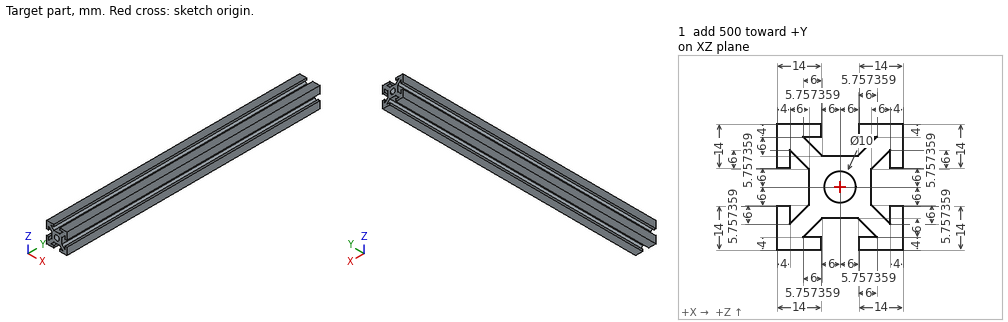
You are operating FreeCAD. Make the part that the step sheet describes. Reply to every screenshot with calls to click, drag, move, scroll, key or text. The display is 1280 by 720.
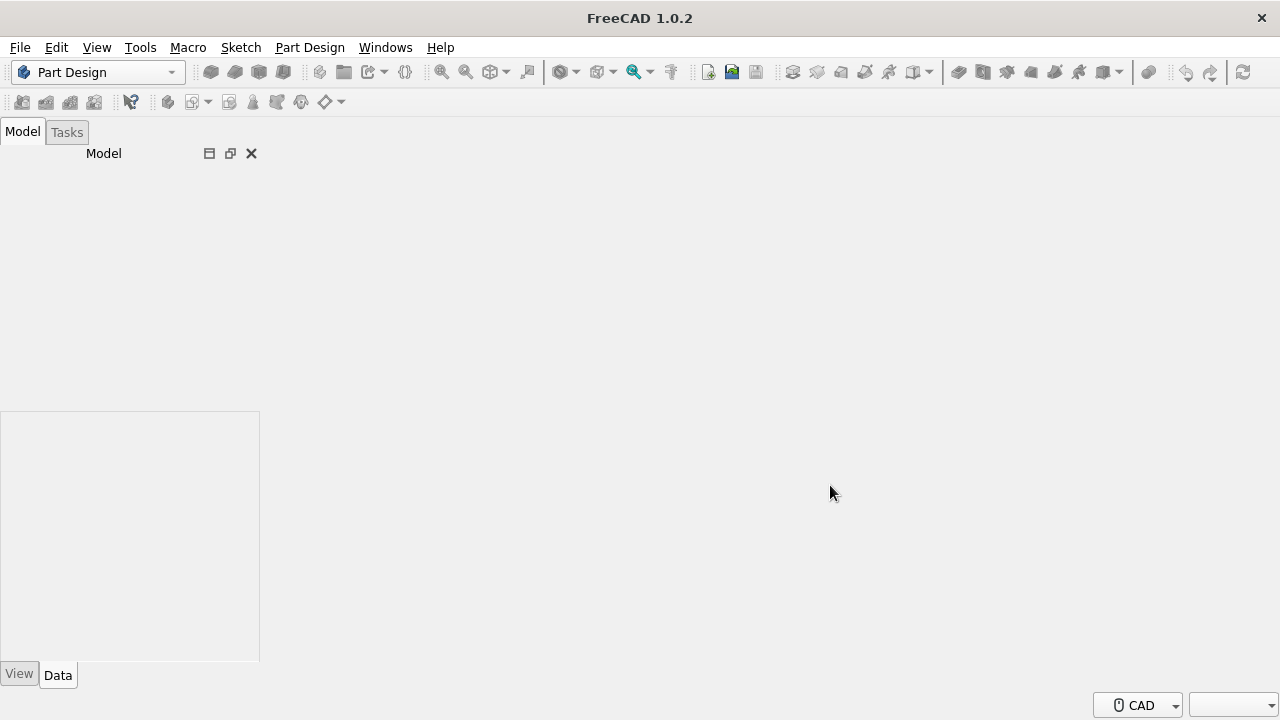
click(708, 72)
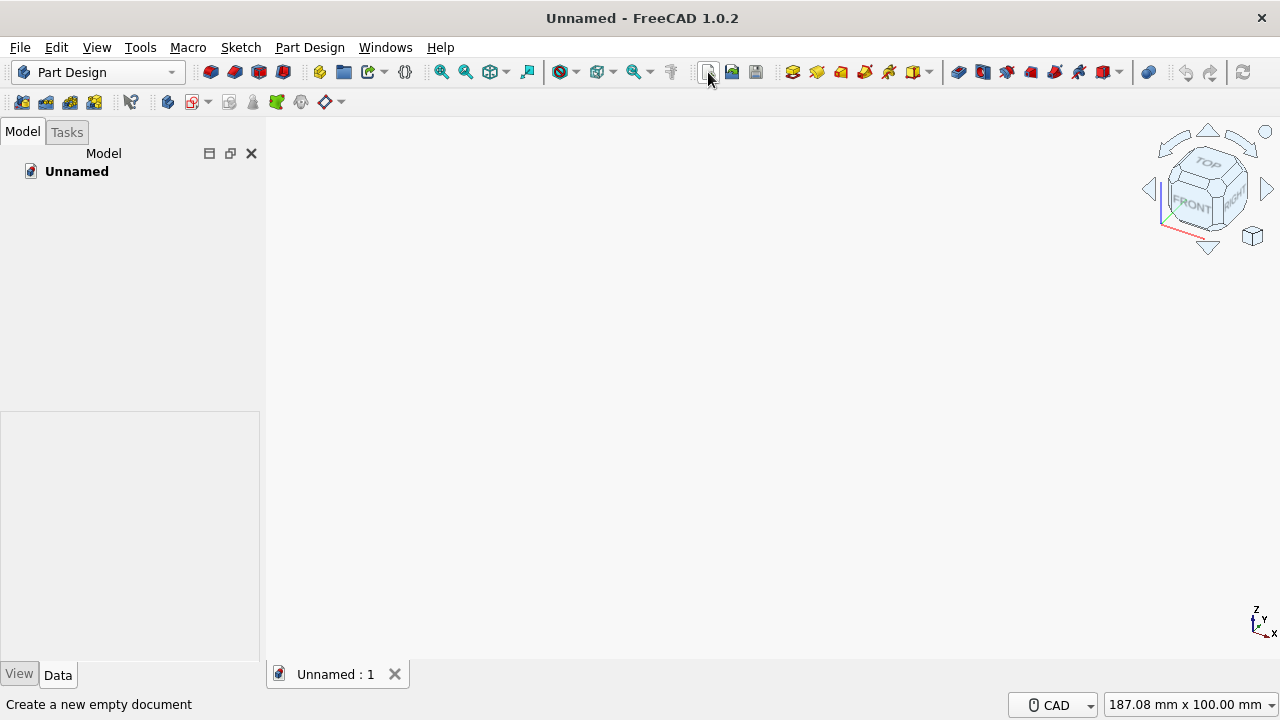
click(192, 102)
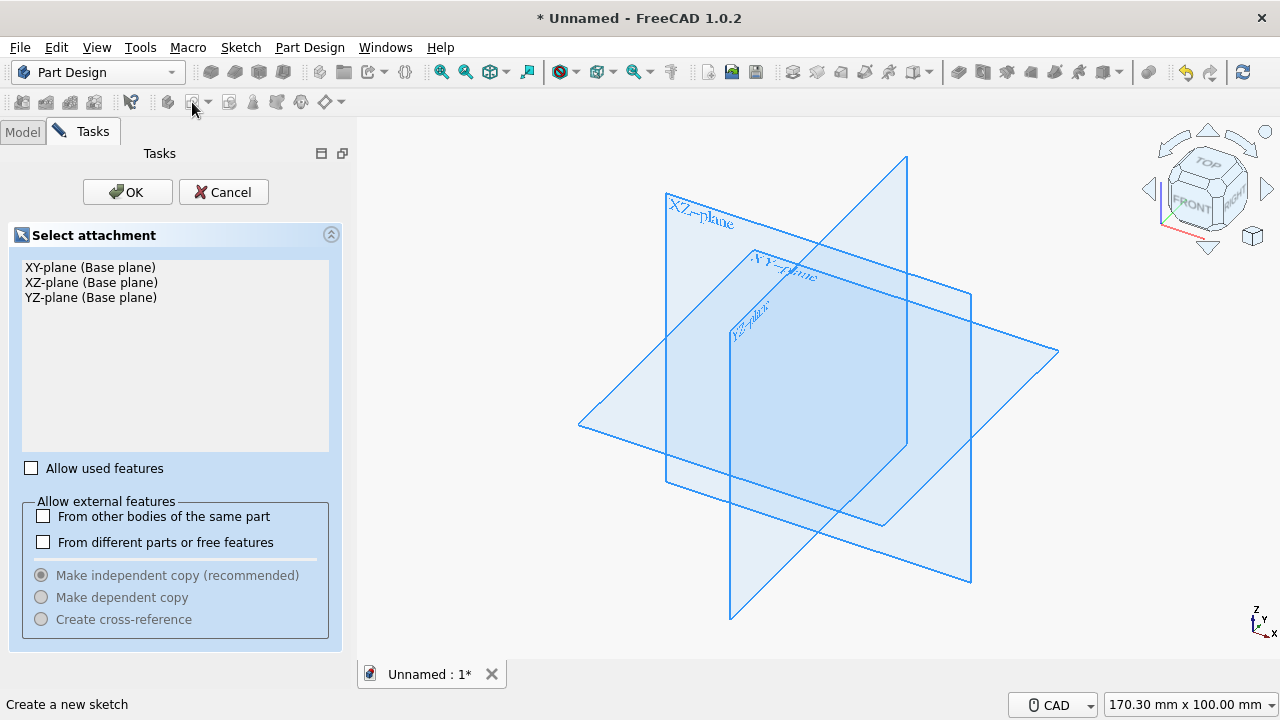
click(82, 282)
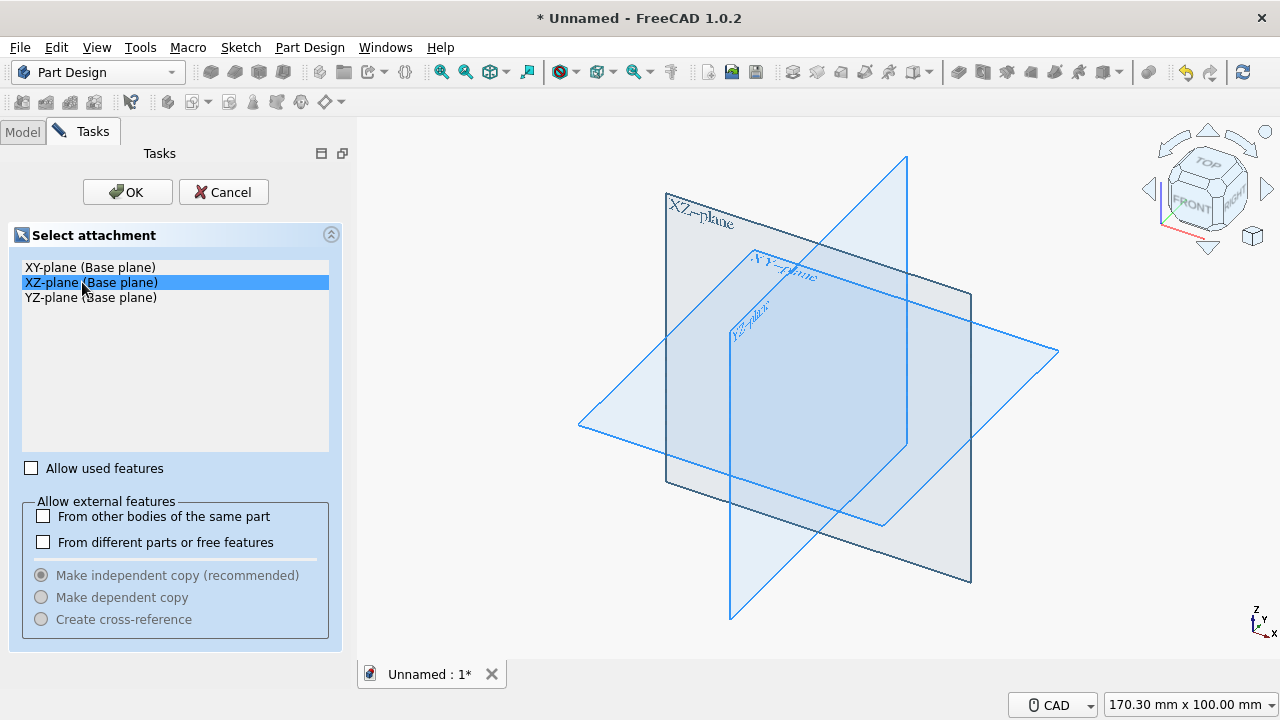
click(128, 192)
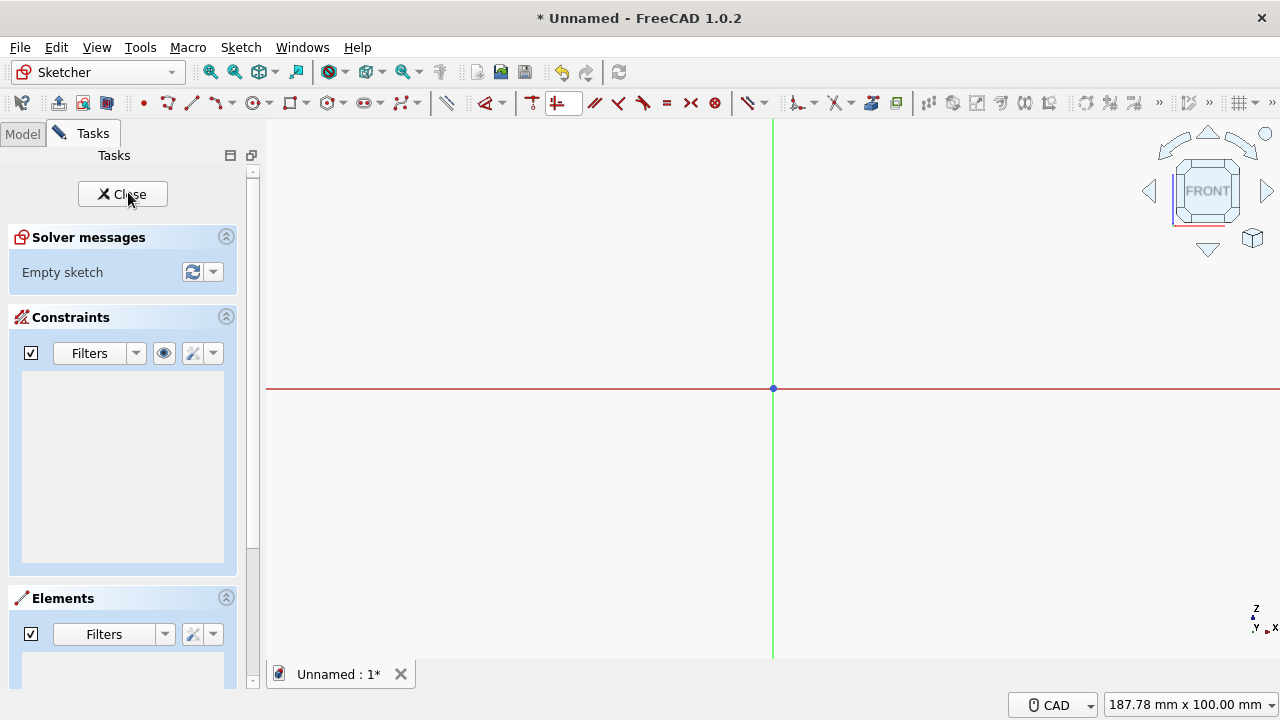
scroll(912, 389, up, 2)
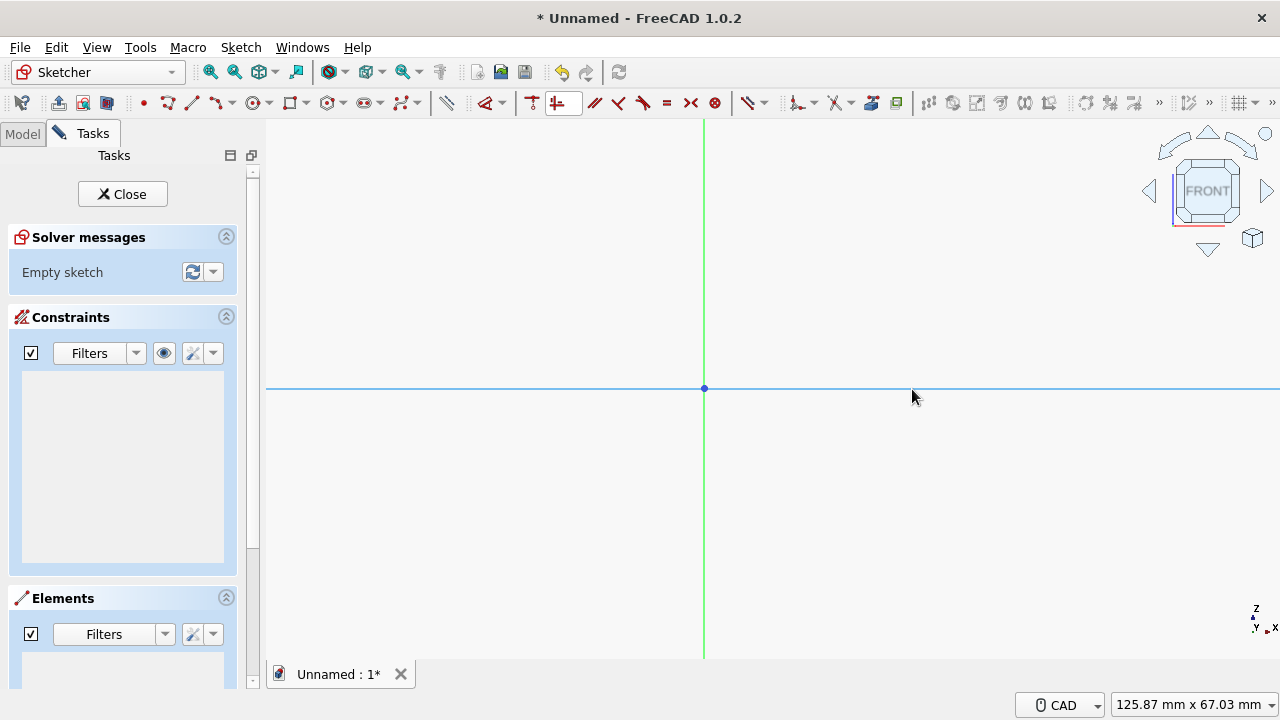
click(168, 104)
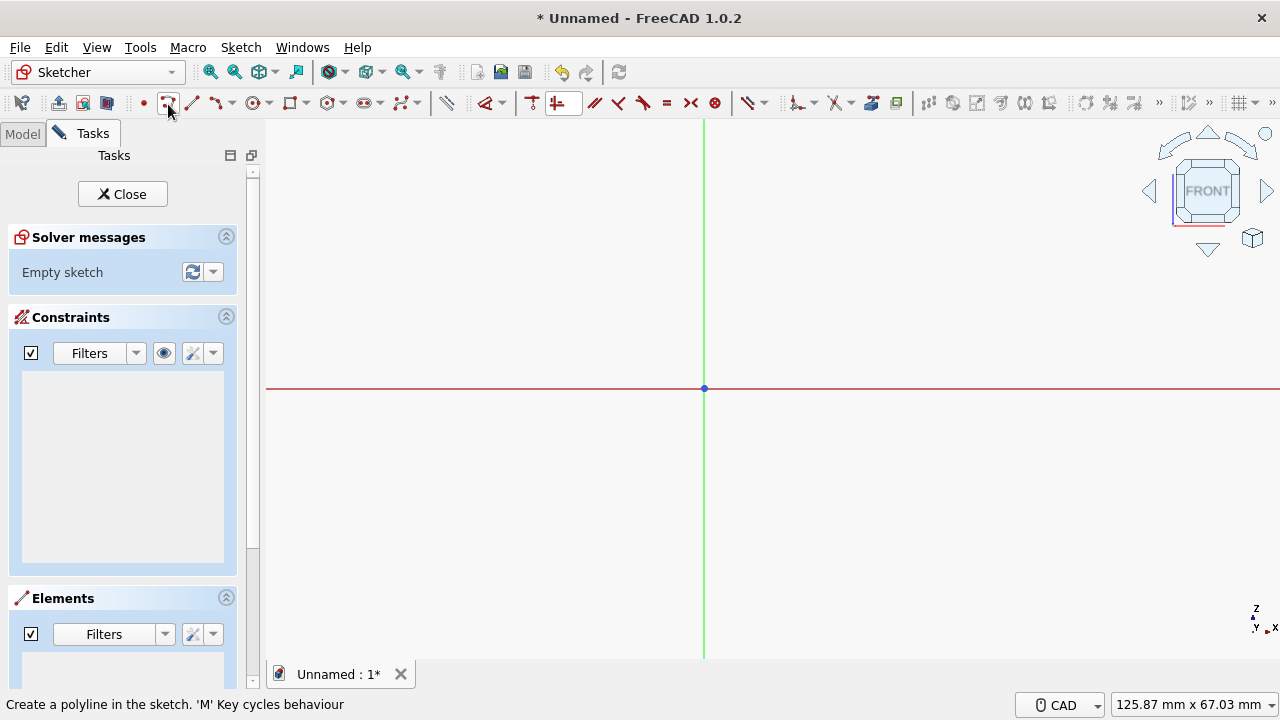
click(624, 435)
click(624, 342)
click(575, 294)
click(575, 340)
click(543, 340)
click(543, 228)
click(656, 228)
click(656, 260)
click(610, 260)
click(658, 308)
click(751, 308)
click(799, 260)
click(753, 260)
click(753, 228)
click(865, 228)
click(865, 340)
click(833, 340)
click(833, 294)
click(785, 342)
click(785, 435)
click(833, 483)
click(833, 437)
click(865, 437)
click(865, 550)
click(753, 550)
click(753, 518)
click(799, 518)
click(751, 469)
click(658, 469)
click(610, 518)
click(656, 518)
click(656, 550)
click(543, 550)
click(543, 437)
click(575, 437)
click(575, 483)
click(624, 436)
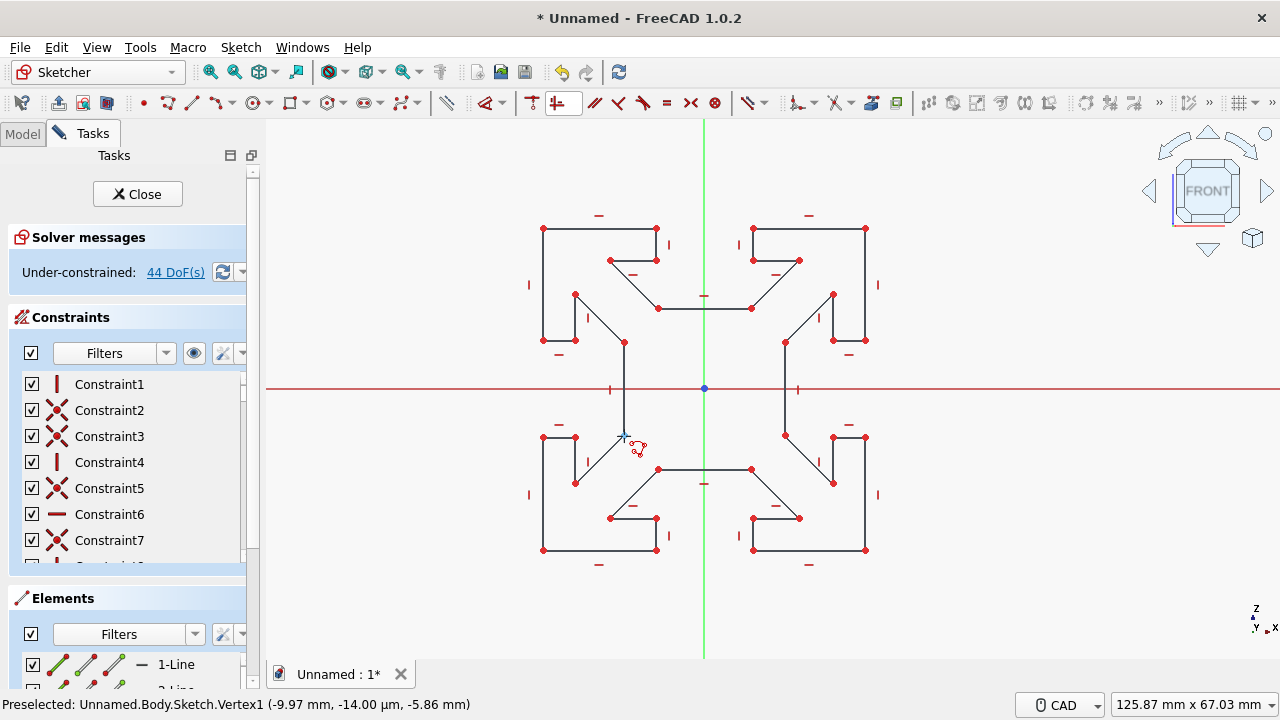
click(254, 104)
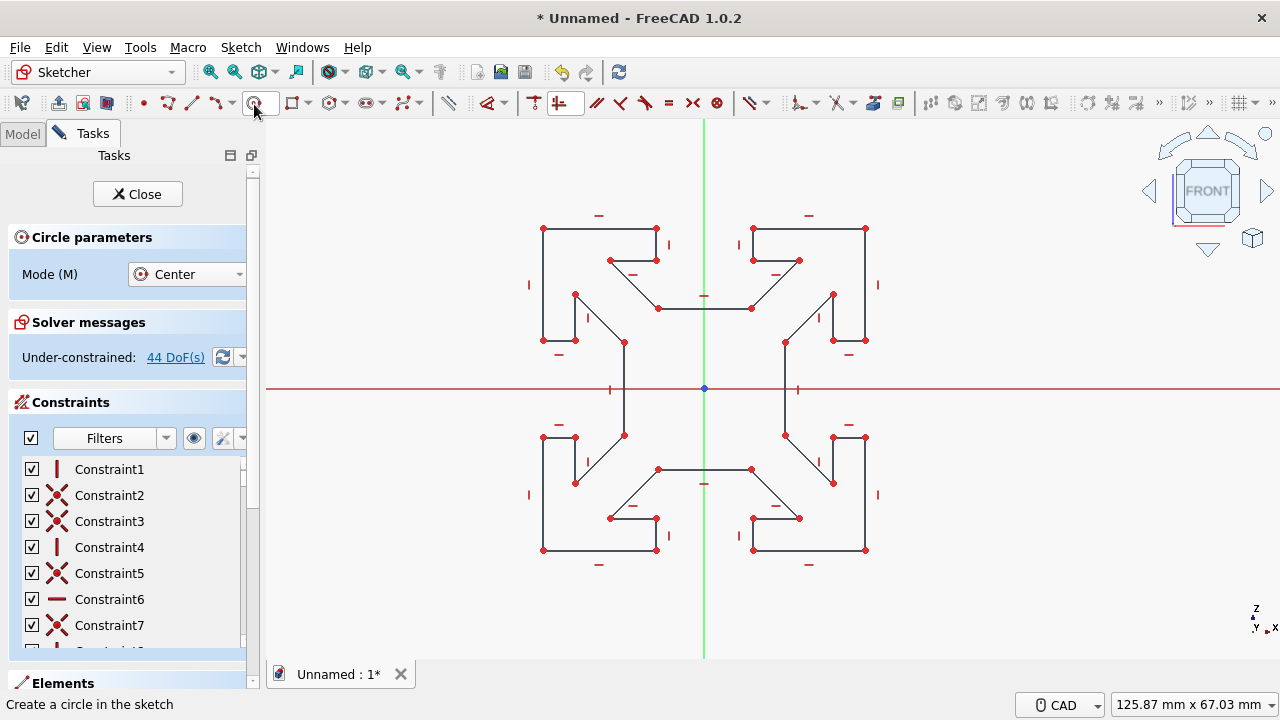
click(704, 389)
click(733, 360)
key(Escape)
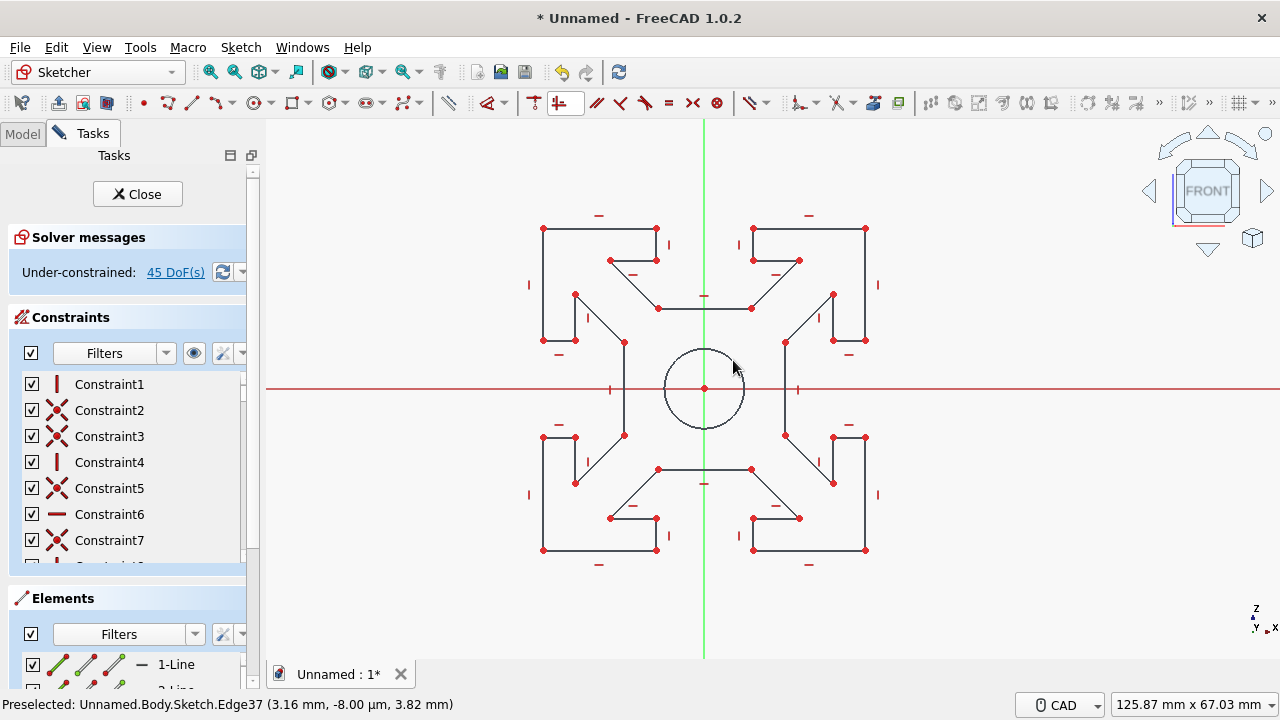
click(488, 104)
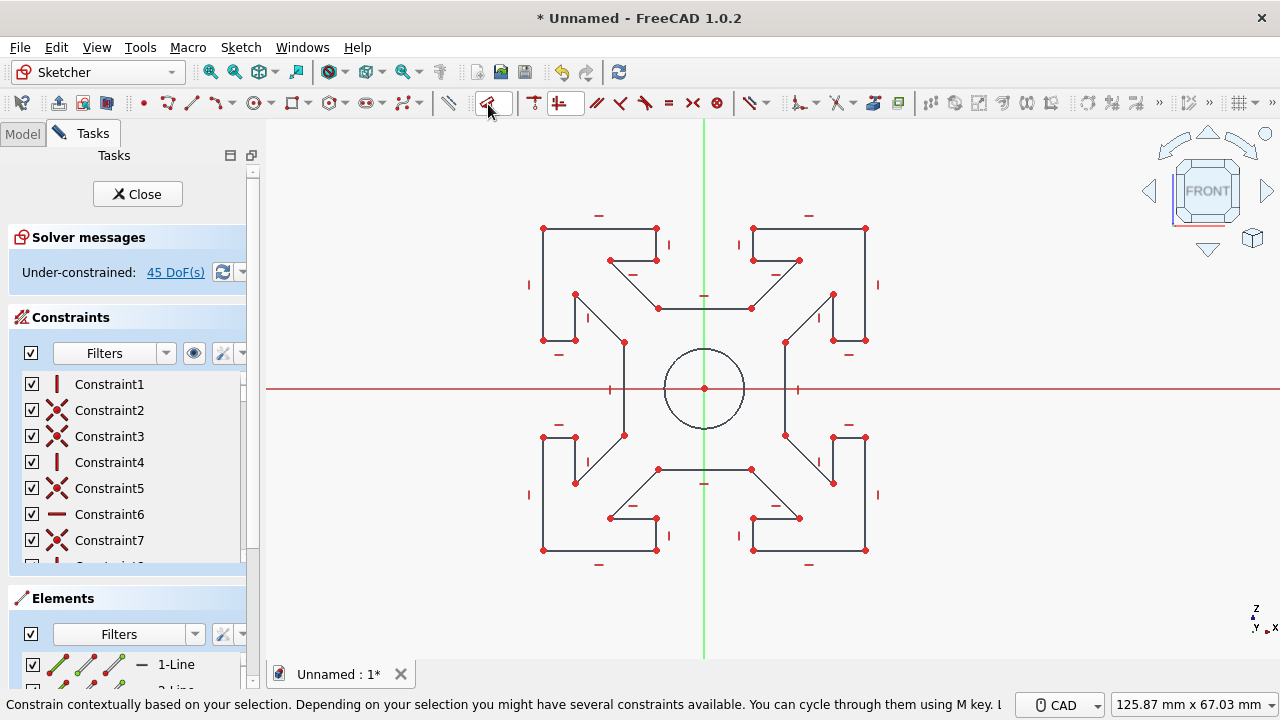
click(732, 360)
click(754, 337)